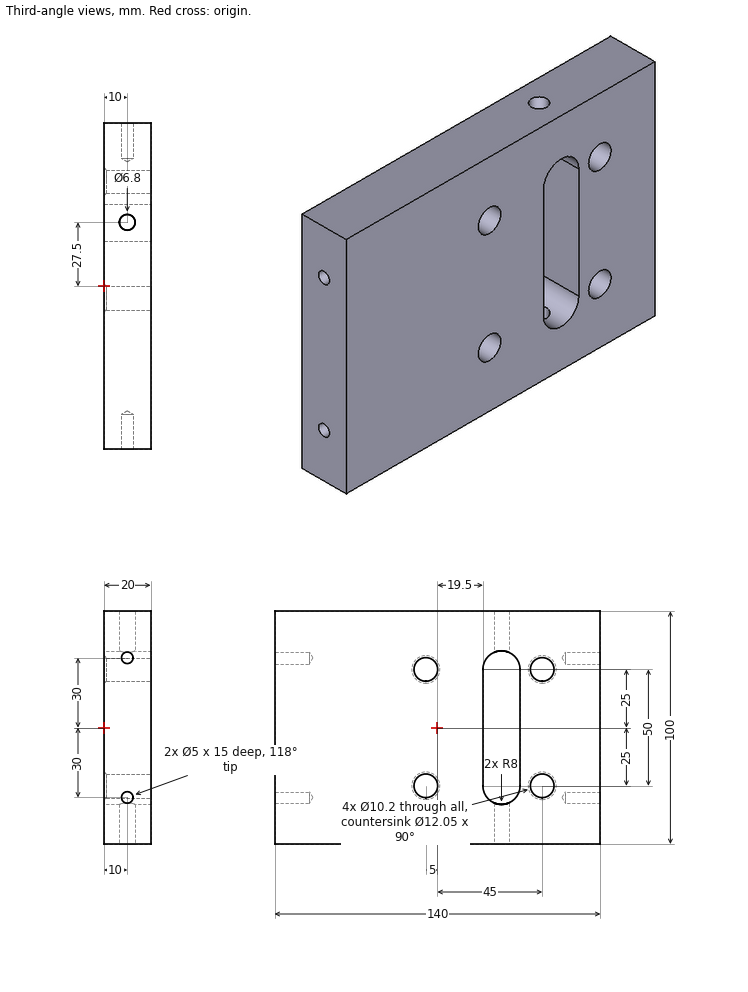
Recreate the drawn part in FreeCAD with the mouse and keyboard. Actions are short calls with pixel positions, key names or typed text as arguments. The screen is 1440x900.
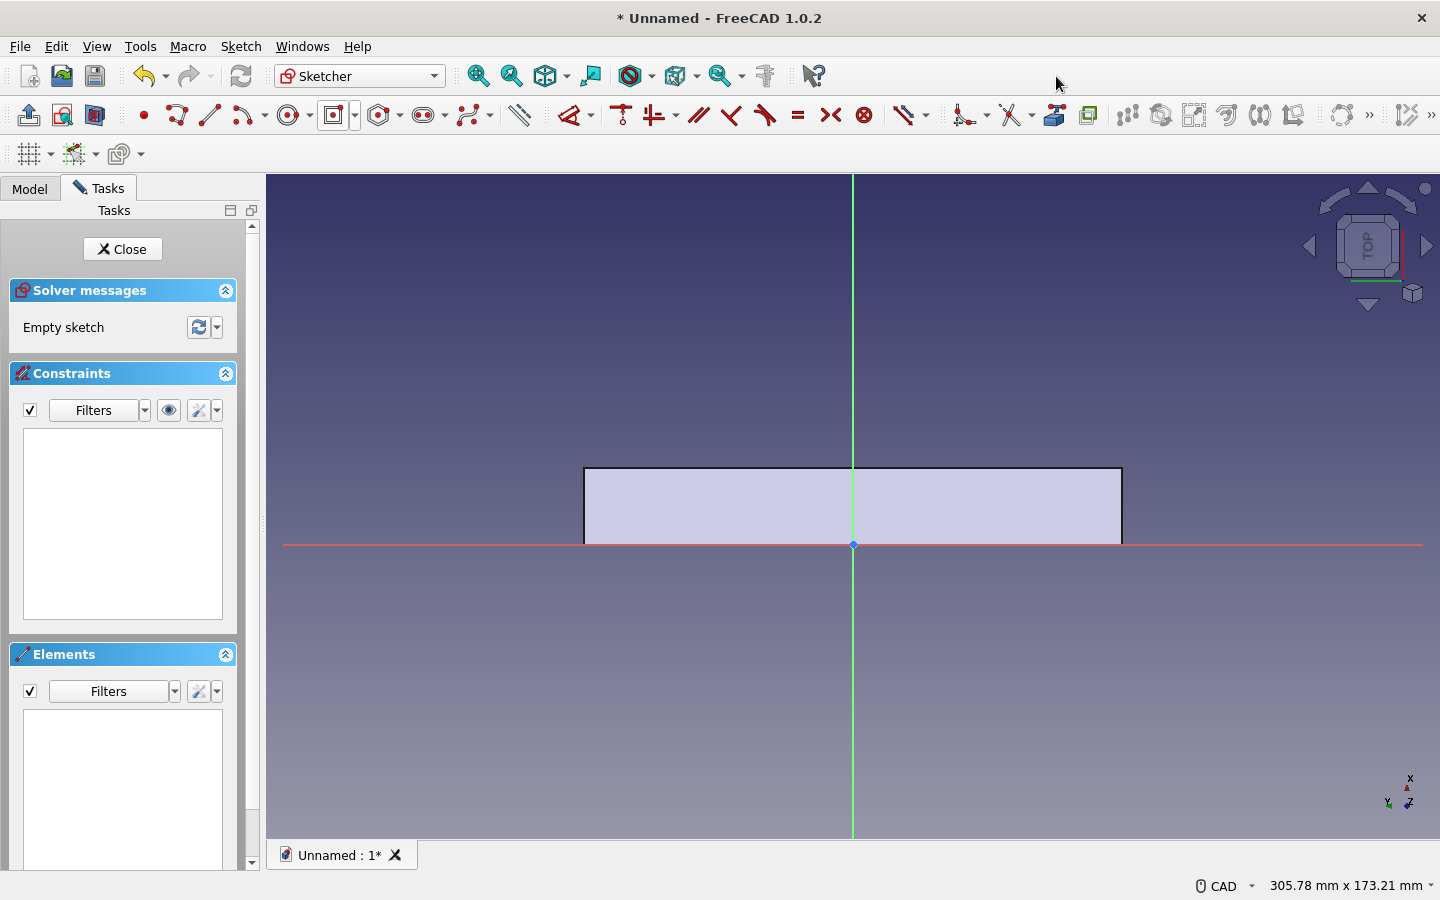
scroll(745, 507, up, 14)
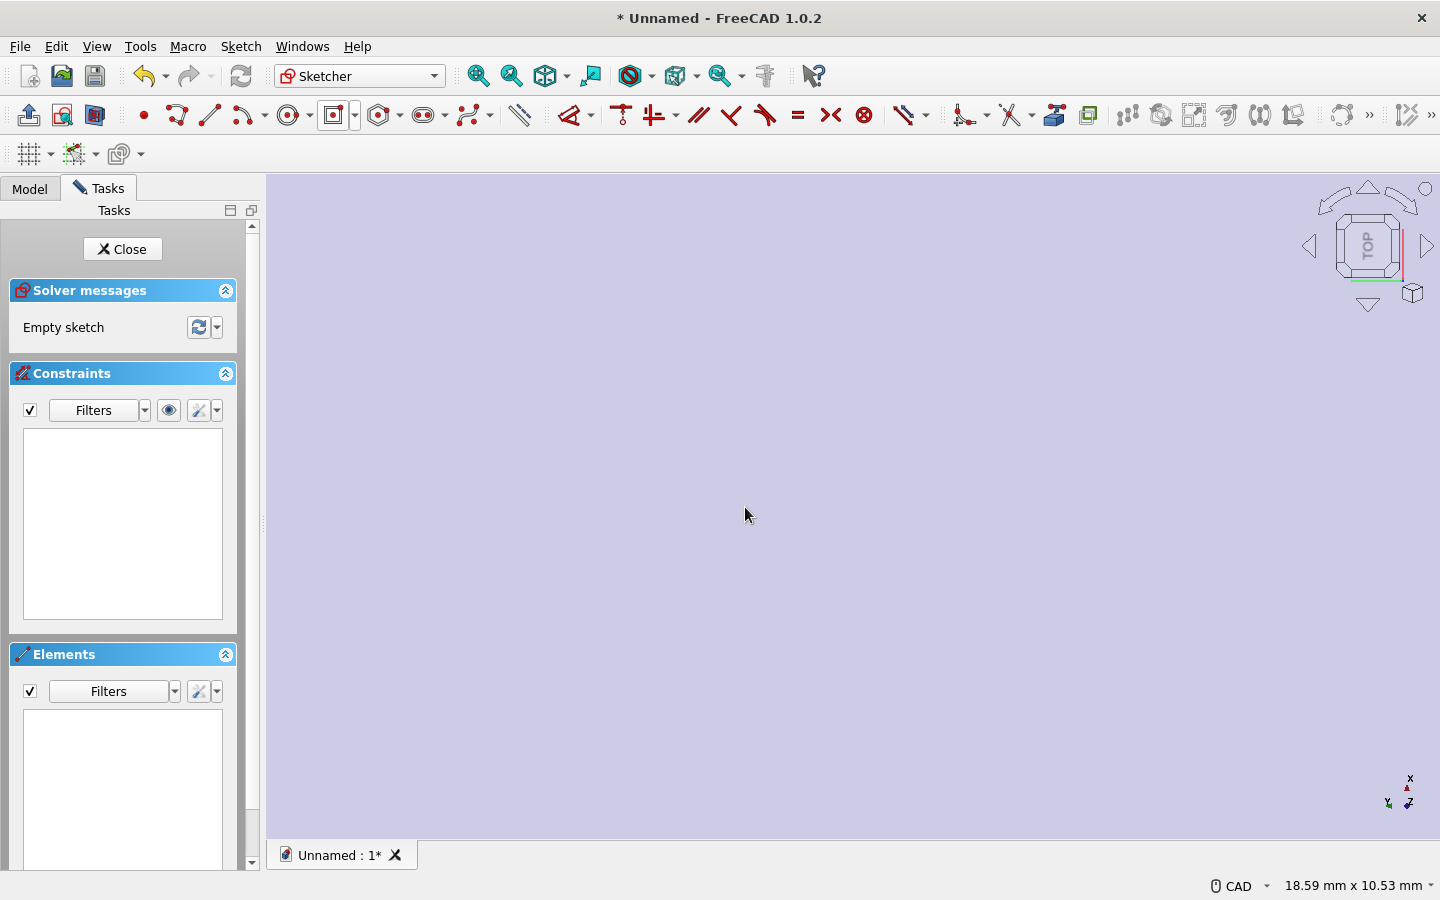
click(288, 116)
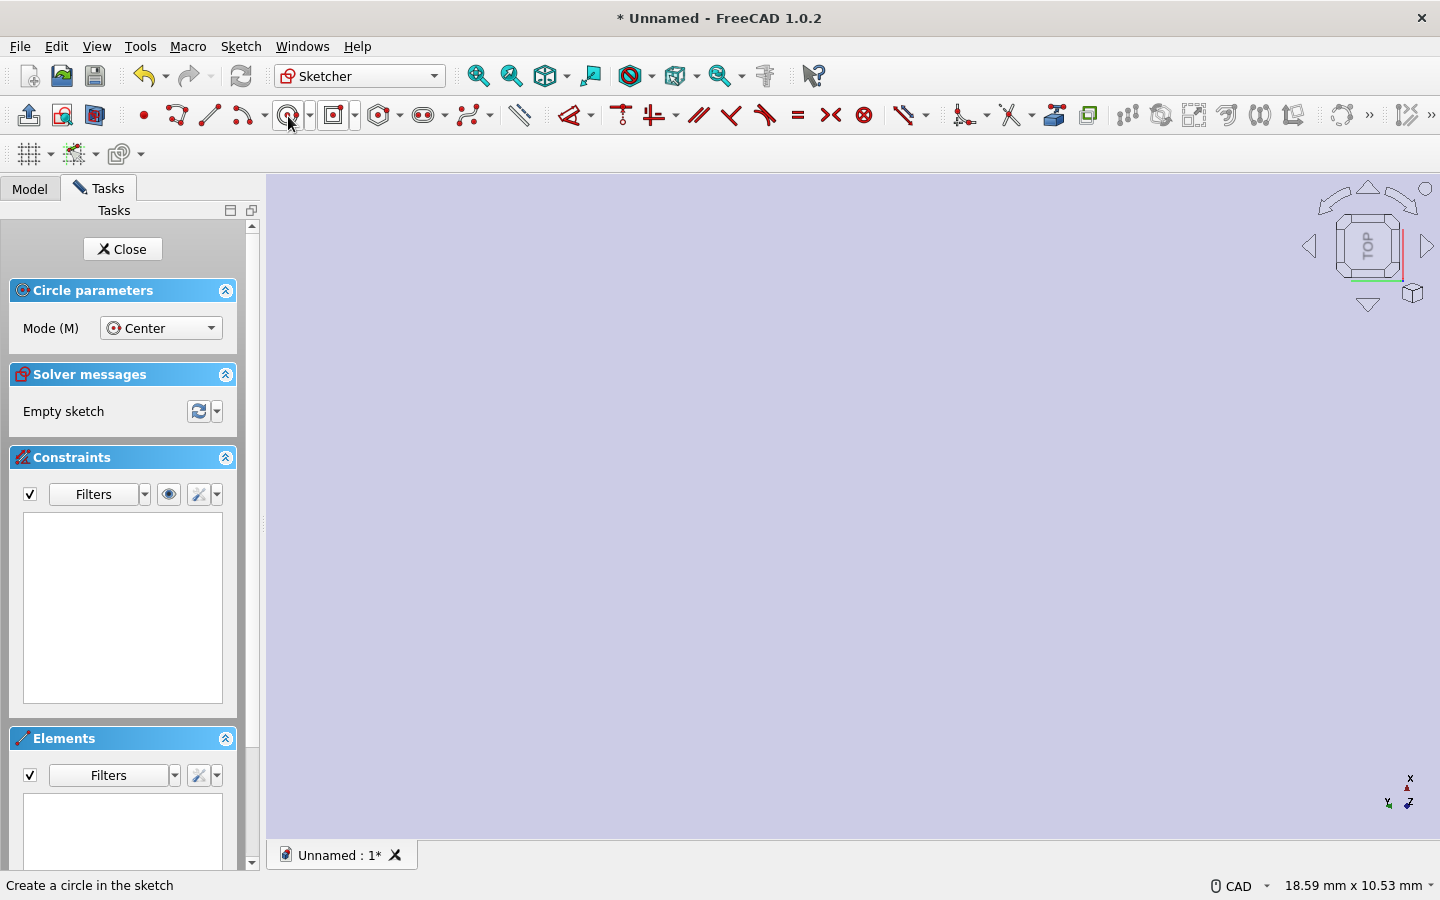
click(778, 491)
move(930, 339)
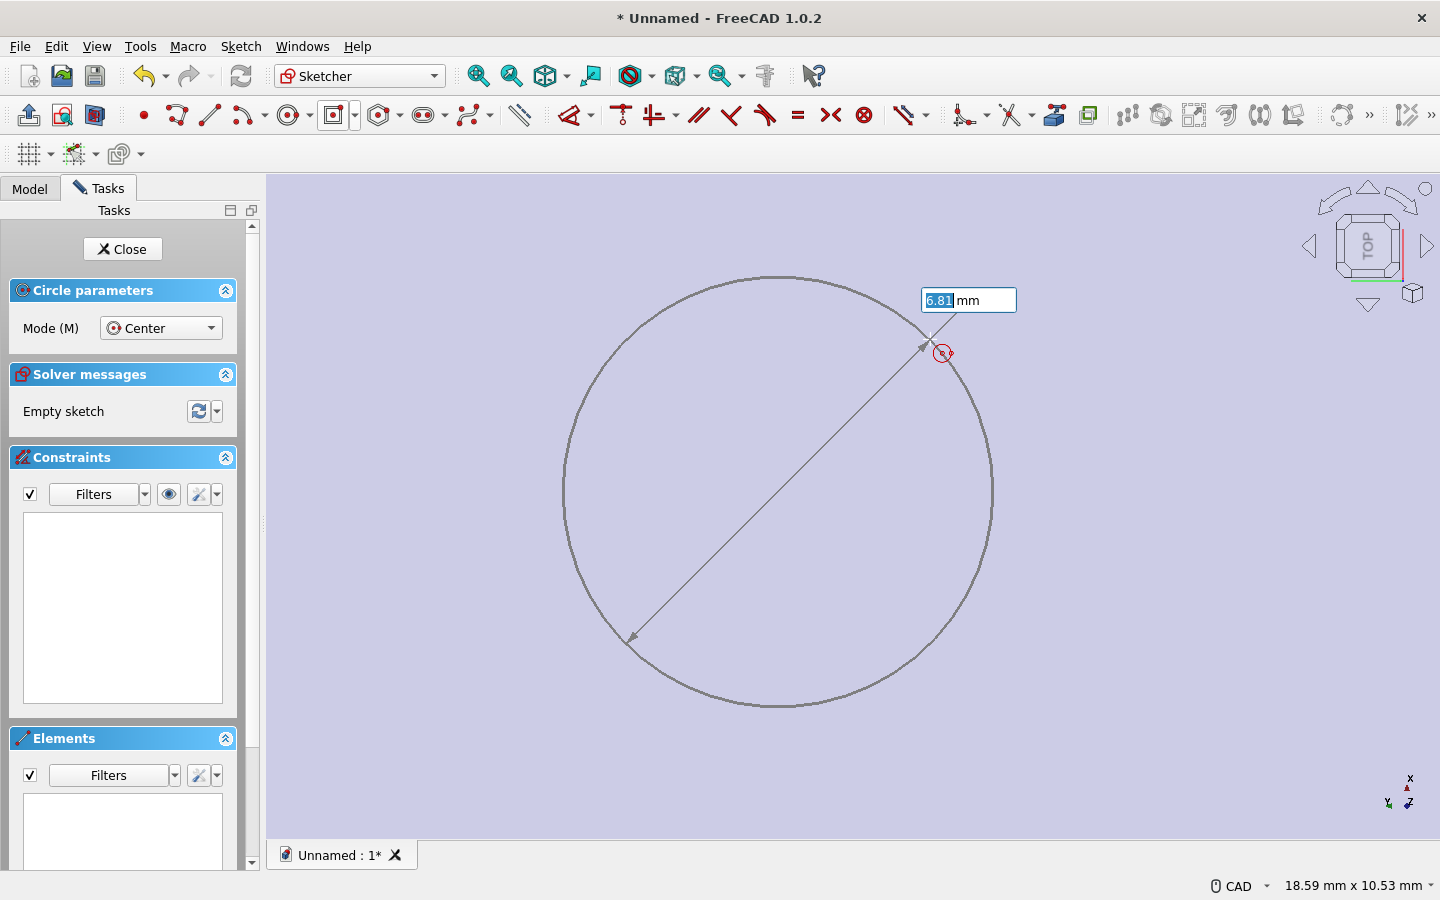
text(6.8)
key(Return)
key(Escape)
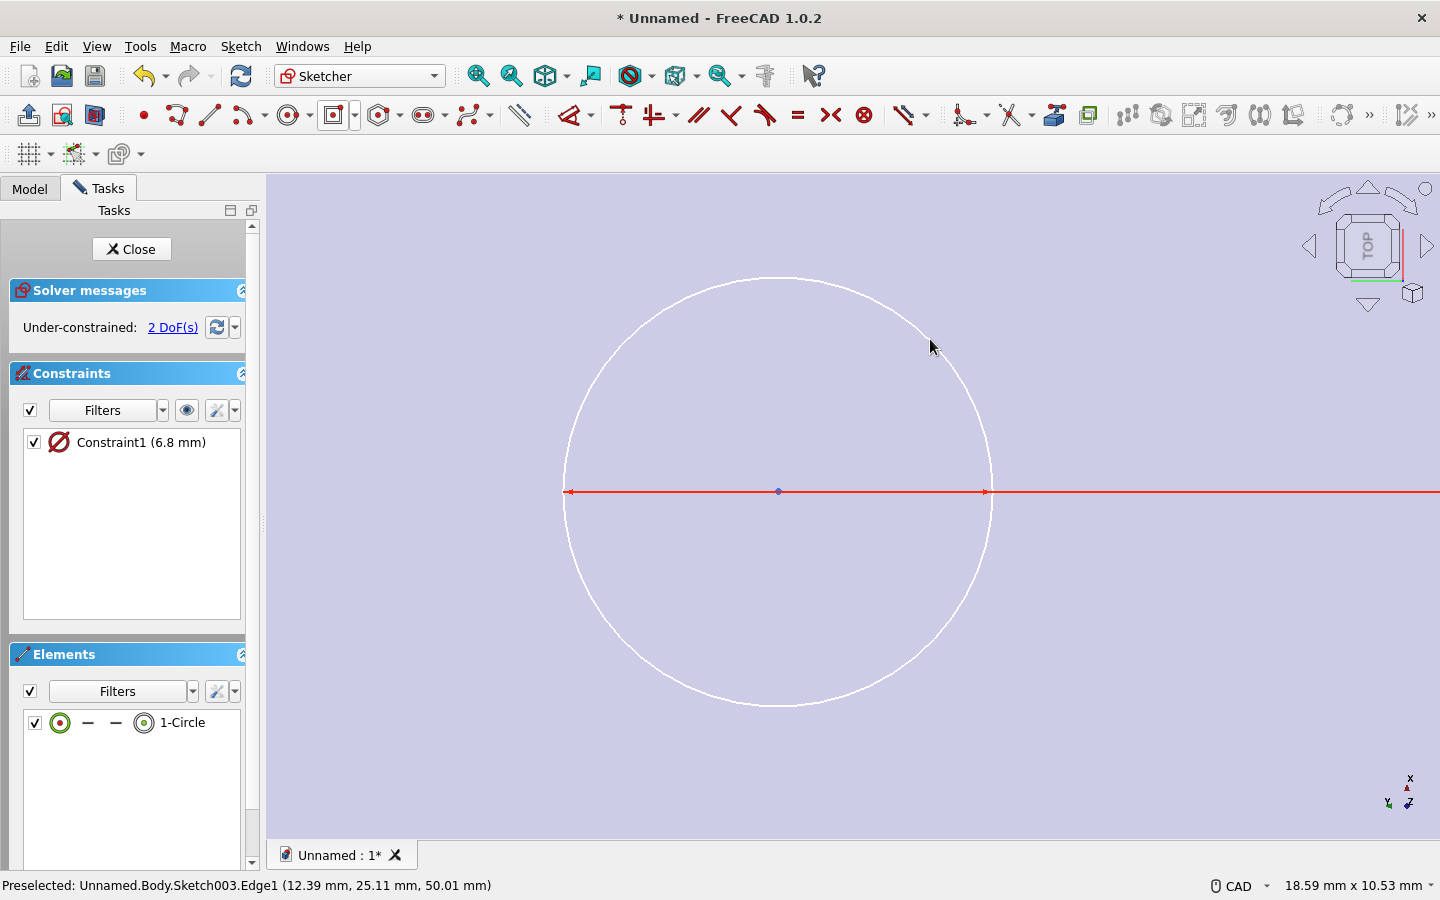
click(568, 116)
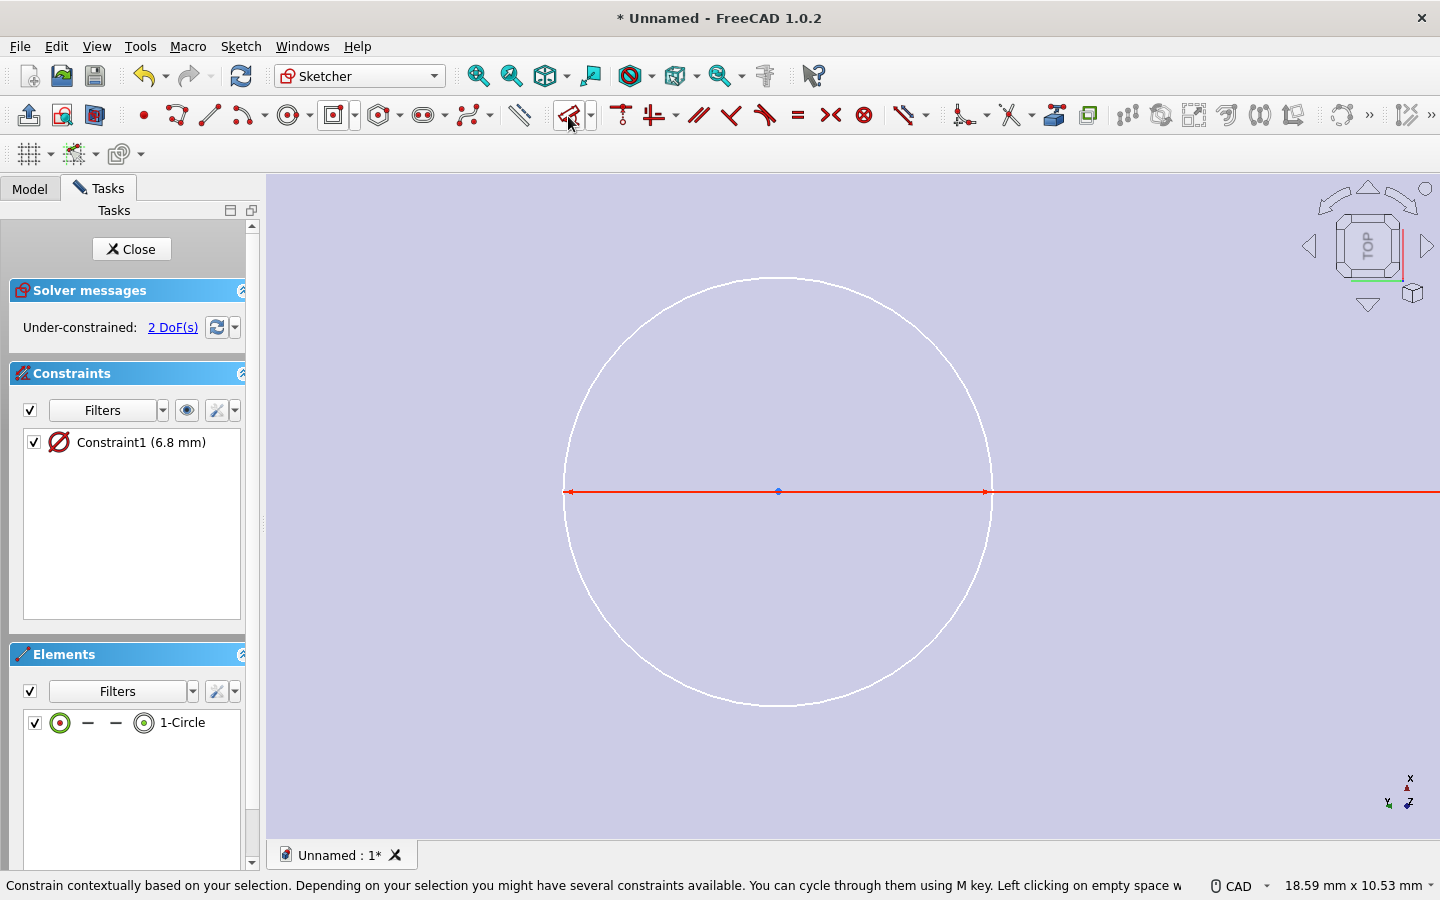
click(778, 492)
click(744, 652)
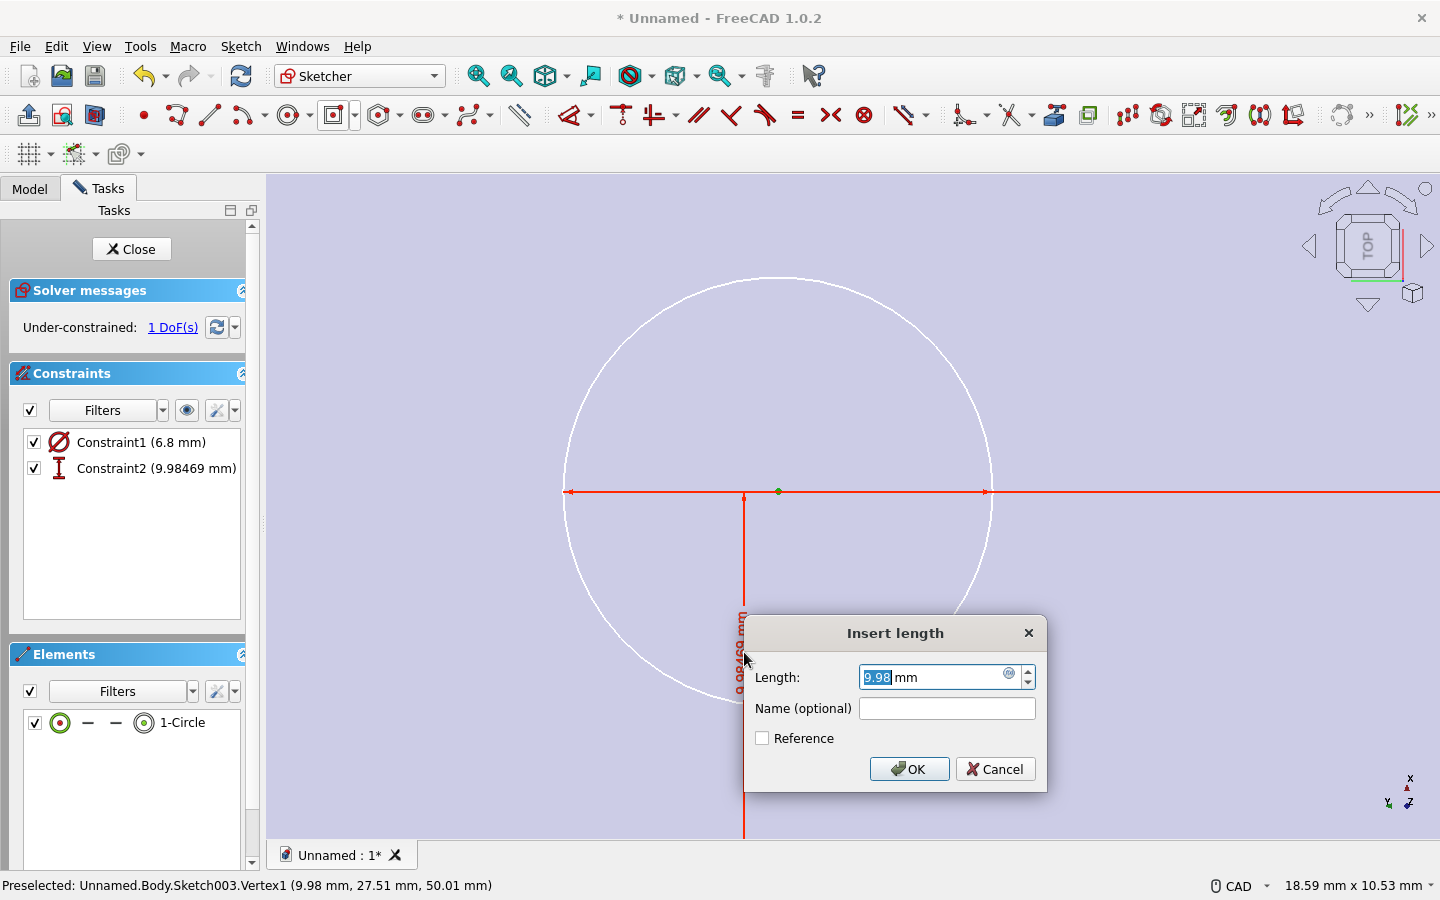
text(10)
key(Return)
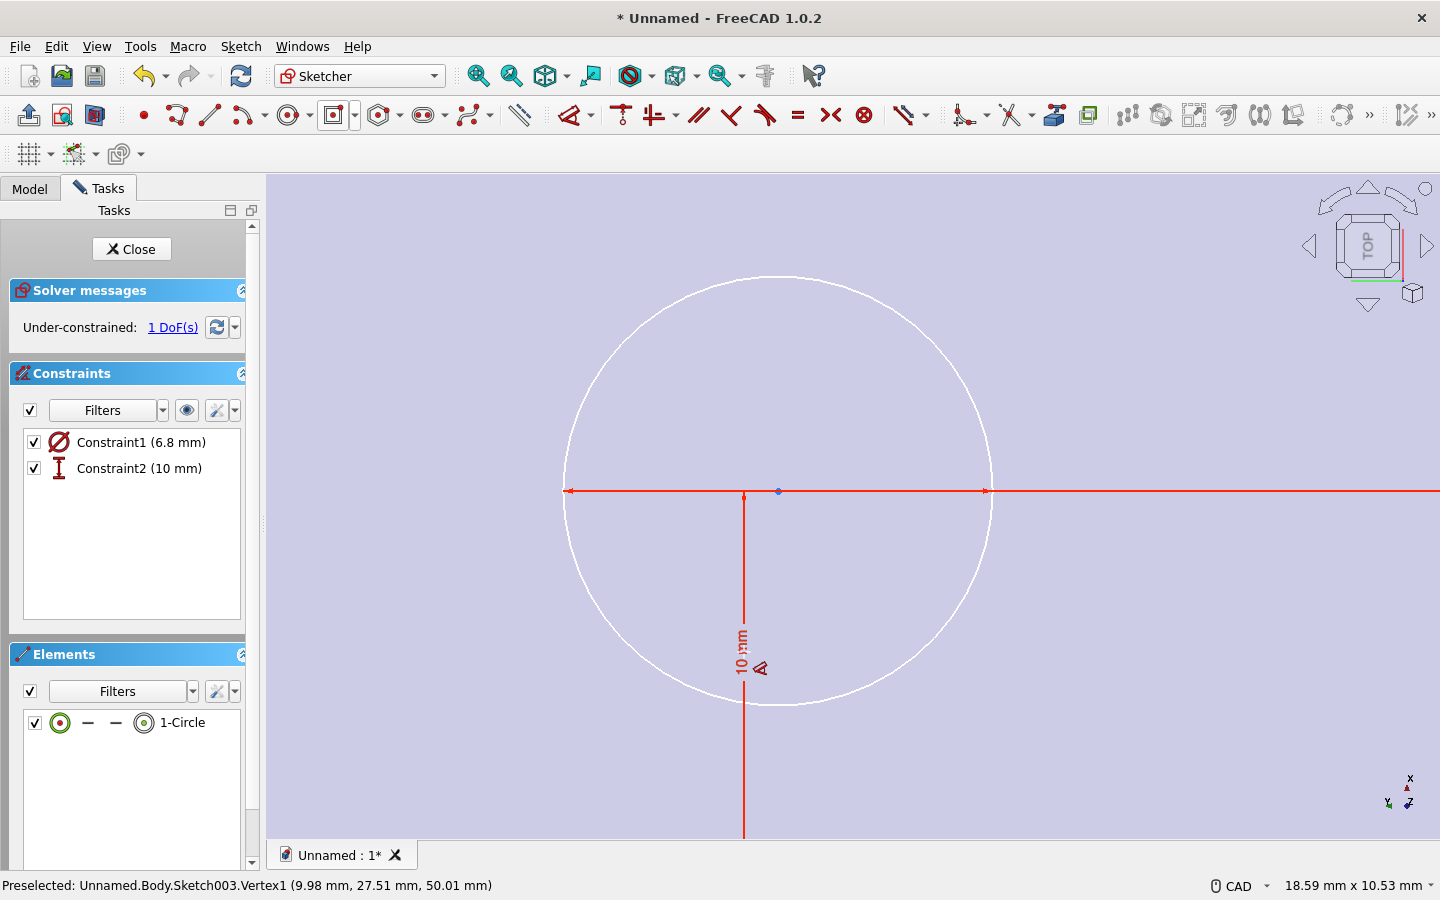
click(778, 491)
click(1027, 457)